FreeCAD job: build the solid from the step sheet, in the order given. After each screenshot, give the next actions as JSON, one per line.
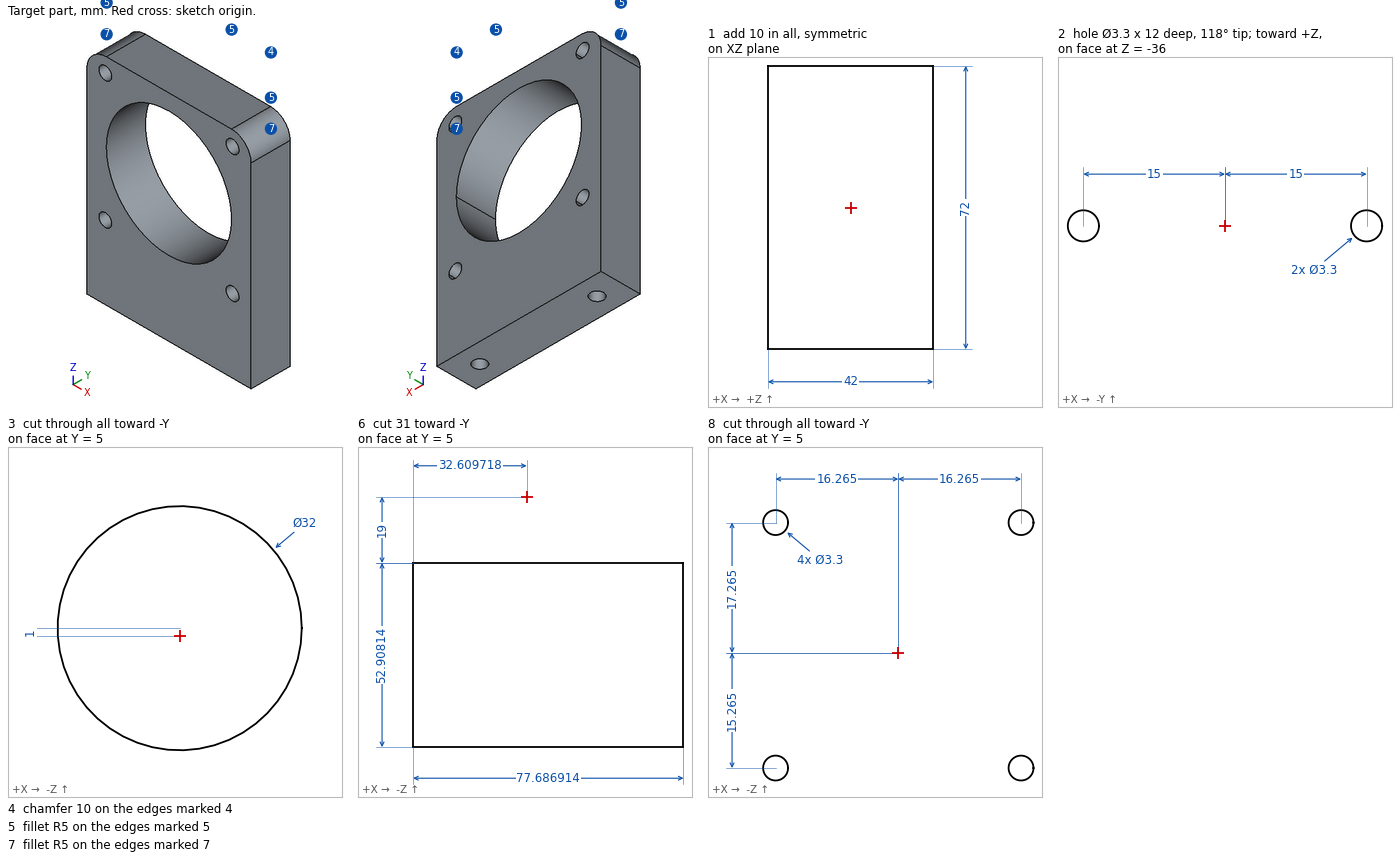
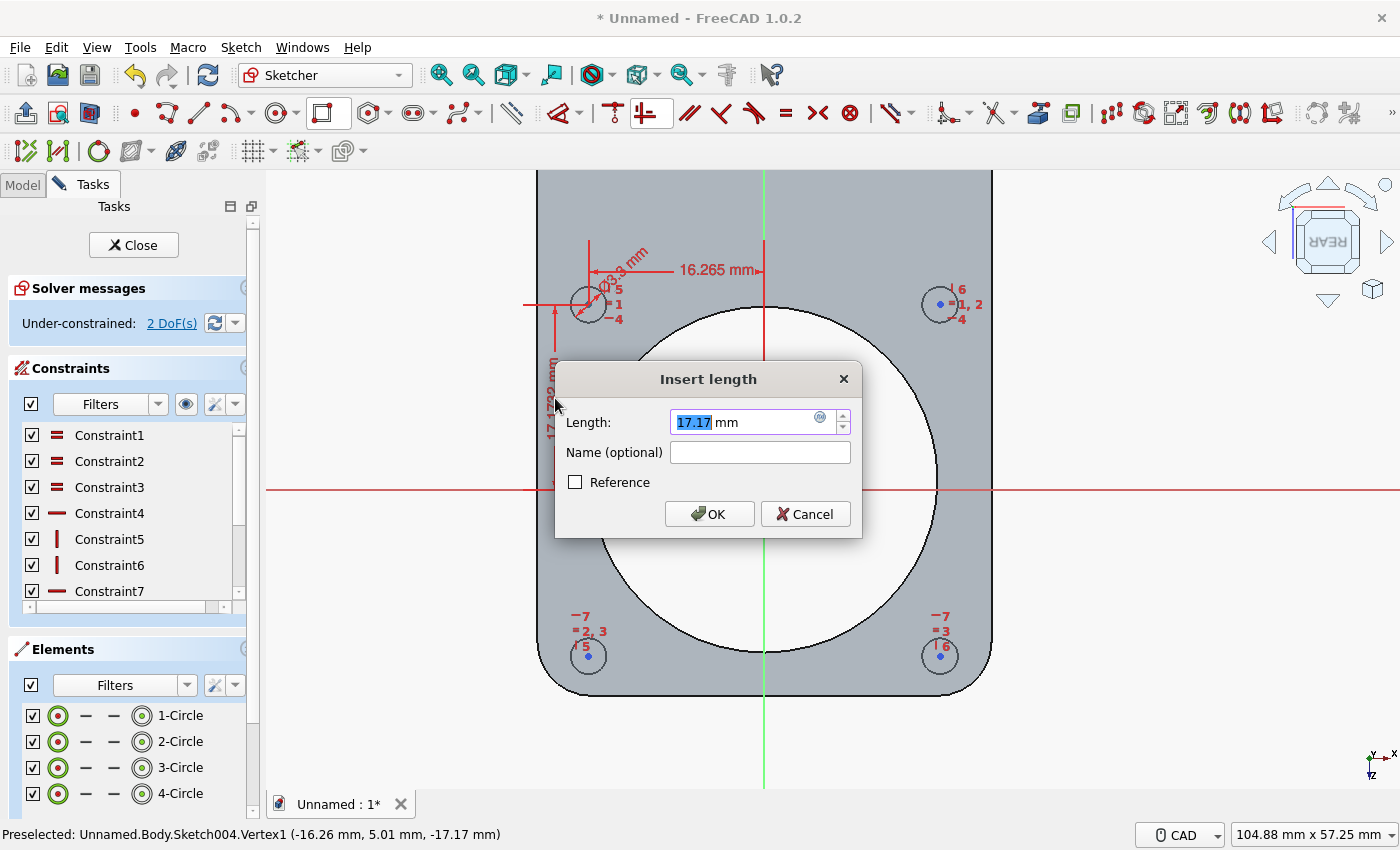
{"action": "type", "text": "17.265"}
{"action": "key", "text": "Return"}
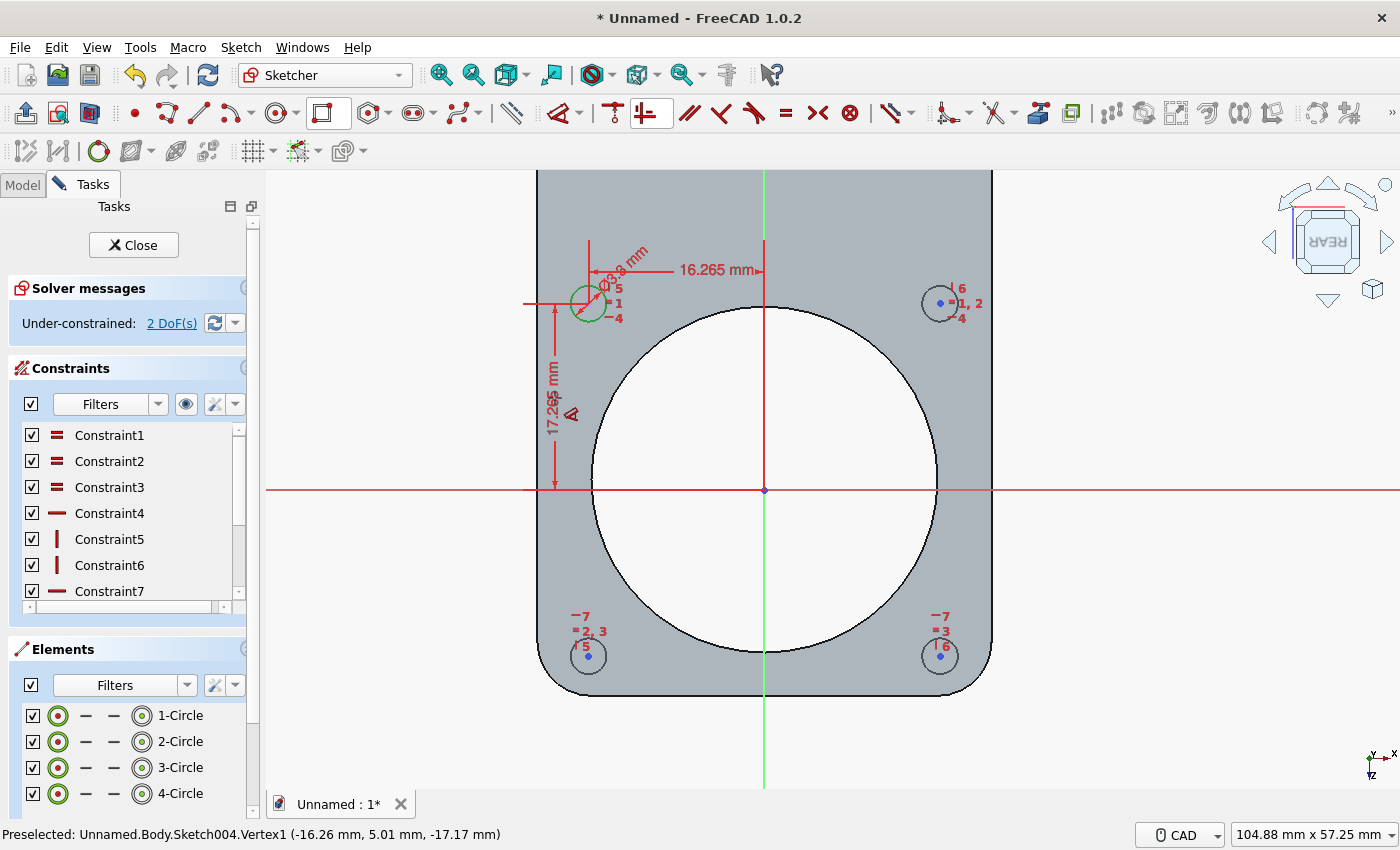
{"action": "left_click", "coordinate": [940, 304]}
{"action": "left_click", "coordinate": [852, 270]}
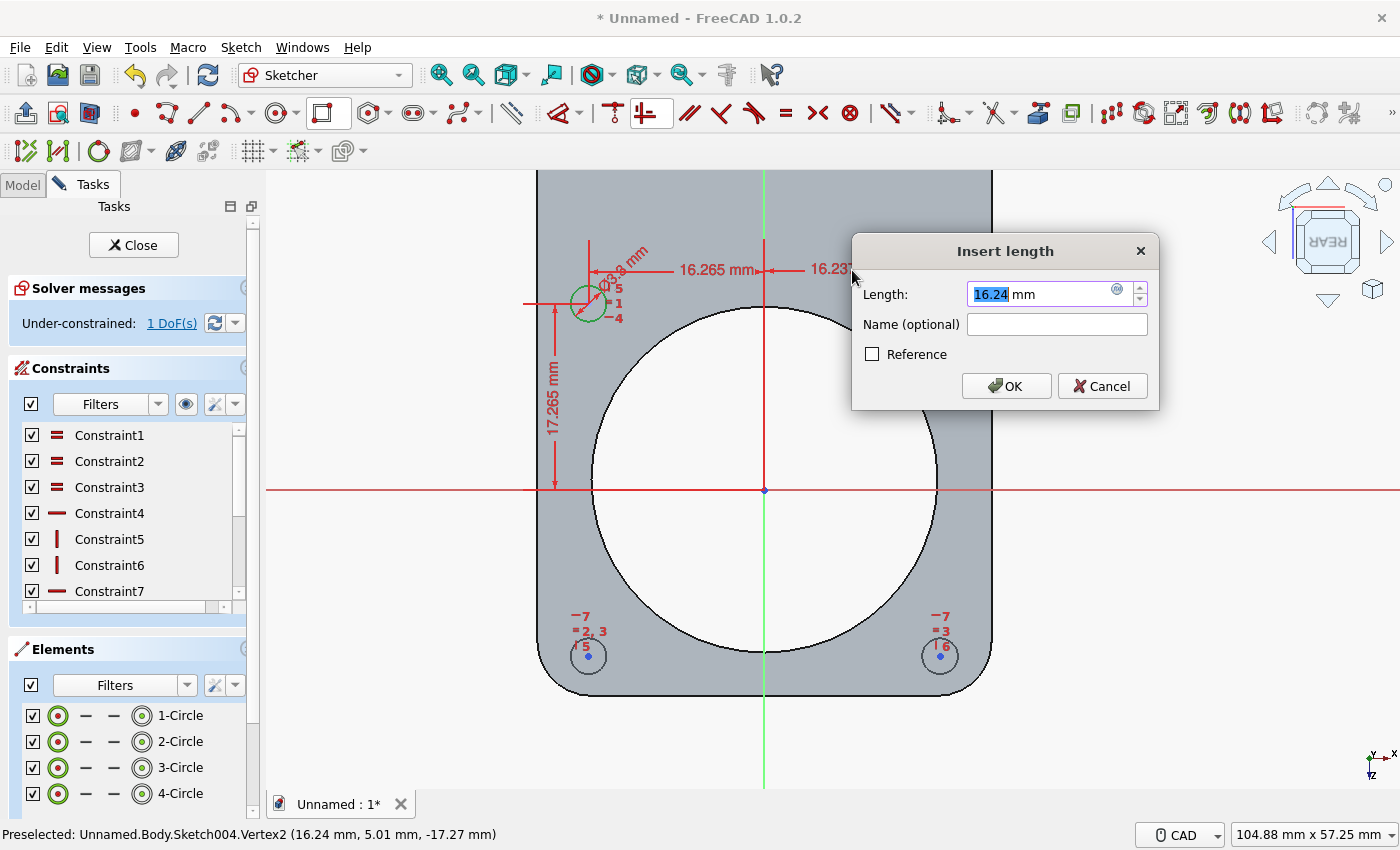
{"action": "type", "text": "16.265"}
{"action": "key", "text": "Return"}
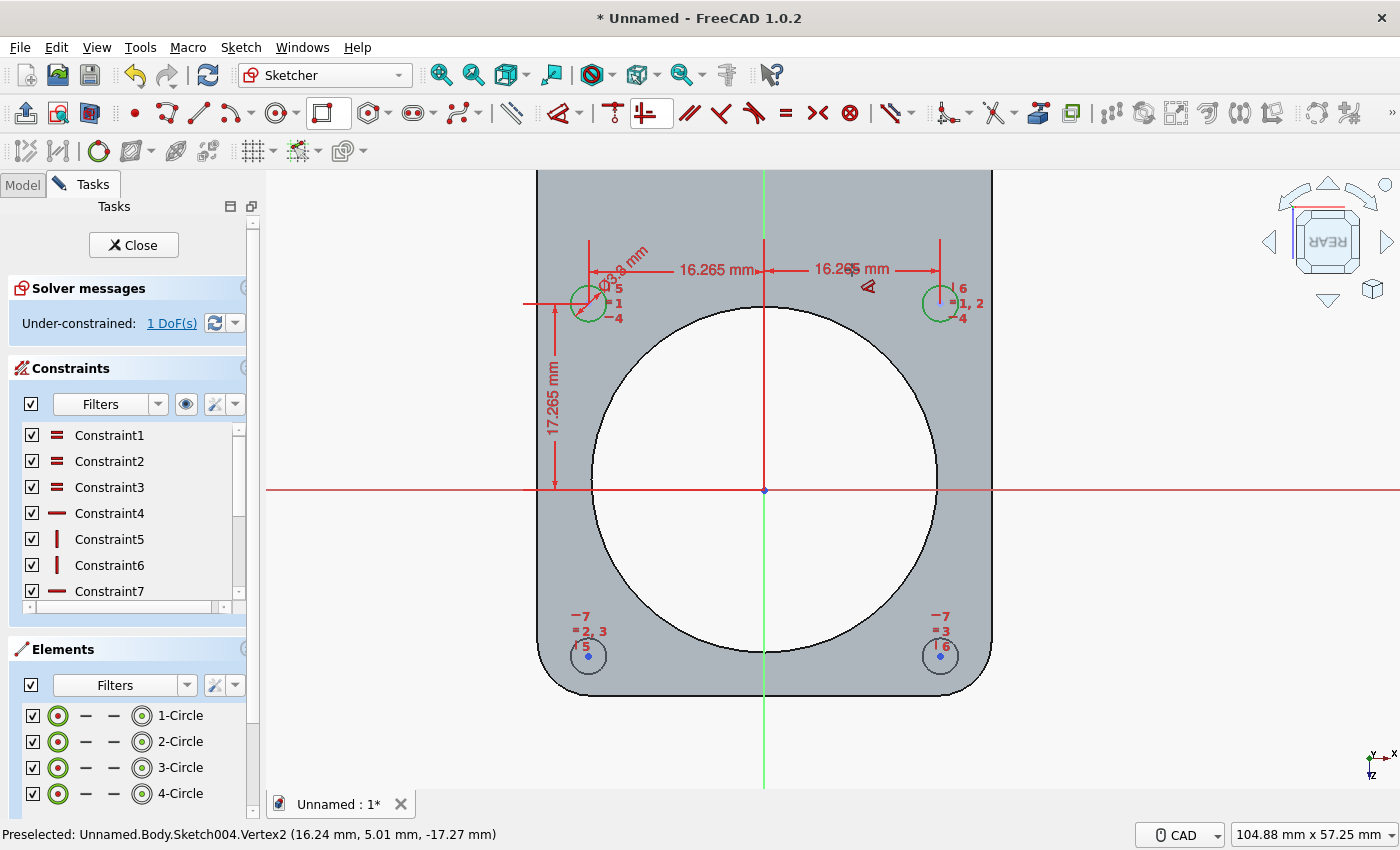
{"action": "left_click", "coordinate": [589, 656]}
{"action": "left_click", "coordinate": [555, 573]}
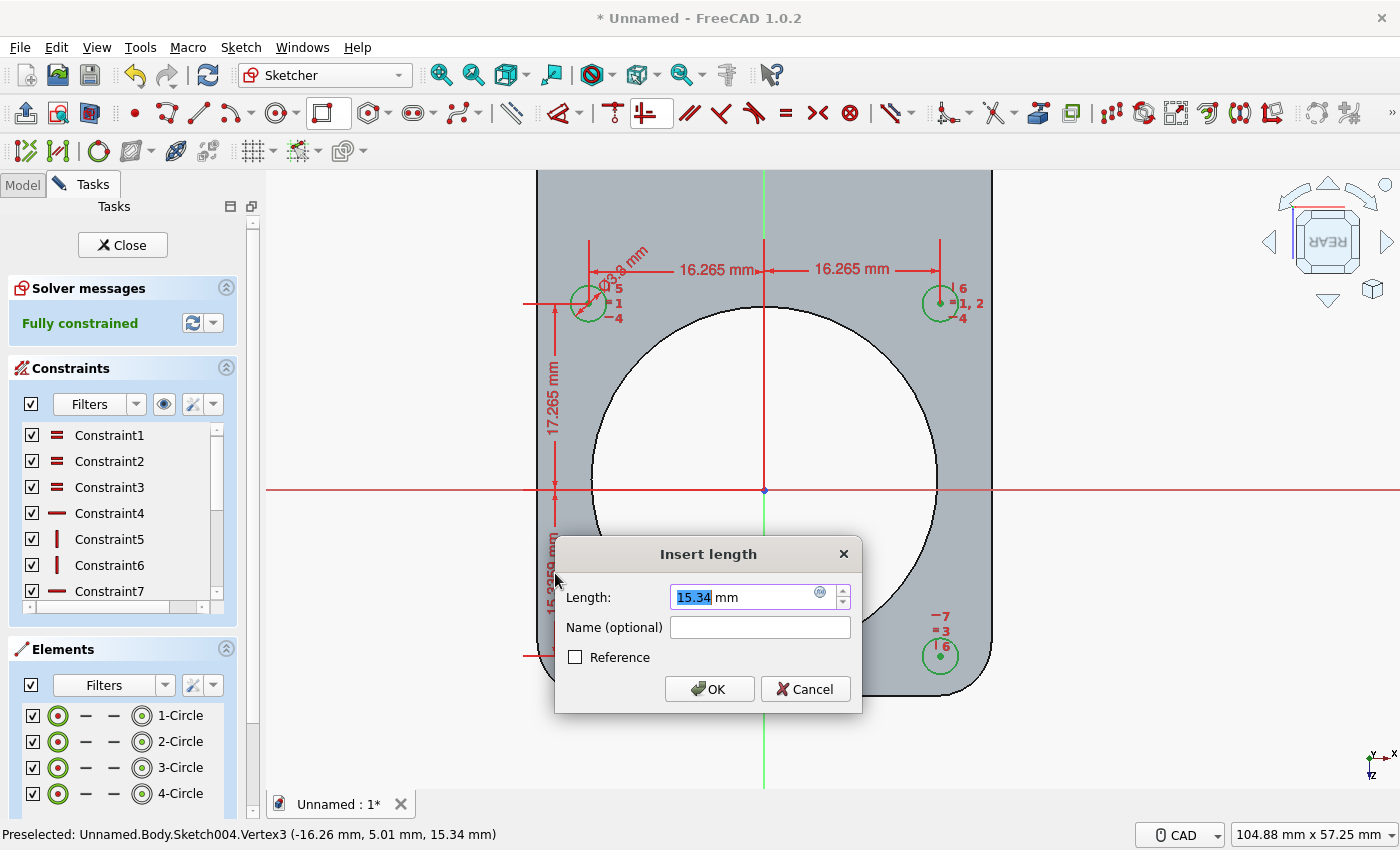
{"action": "type", "text": "15.265"}
{"action": "key", "text": "Return"}
{"action": "key", "text": "Escape"}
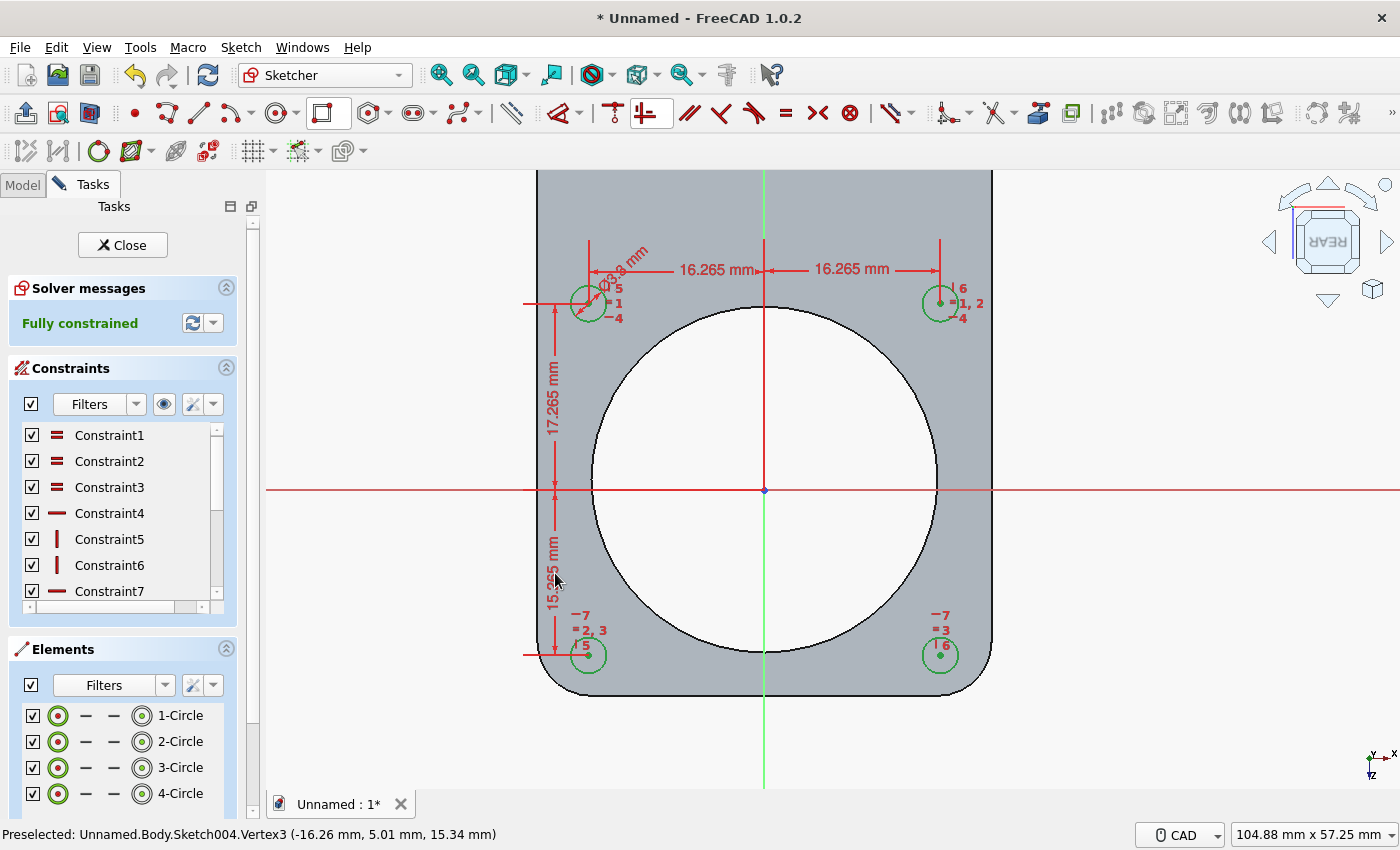
{"action": "left_click", "coordinate": [123, 245]}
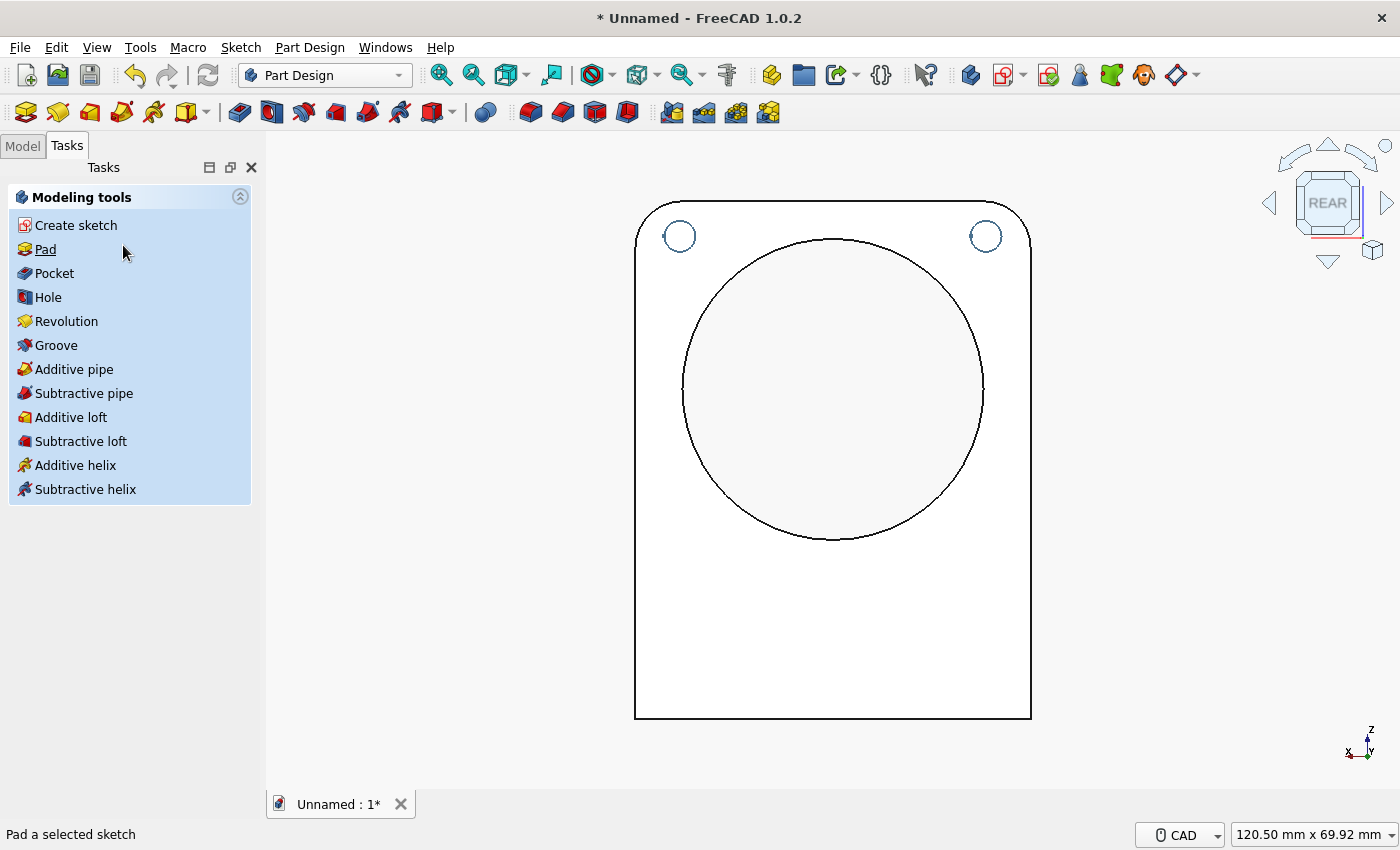
{"action": "left_click", "coordinate": [240, 112]}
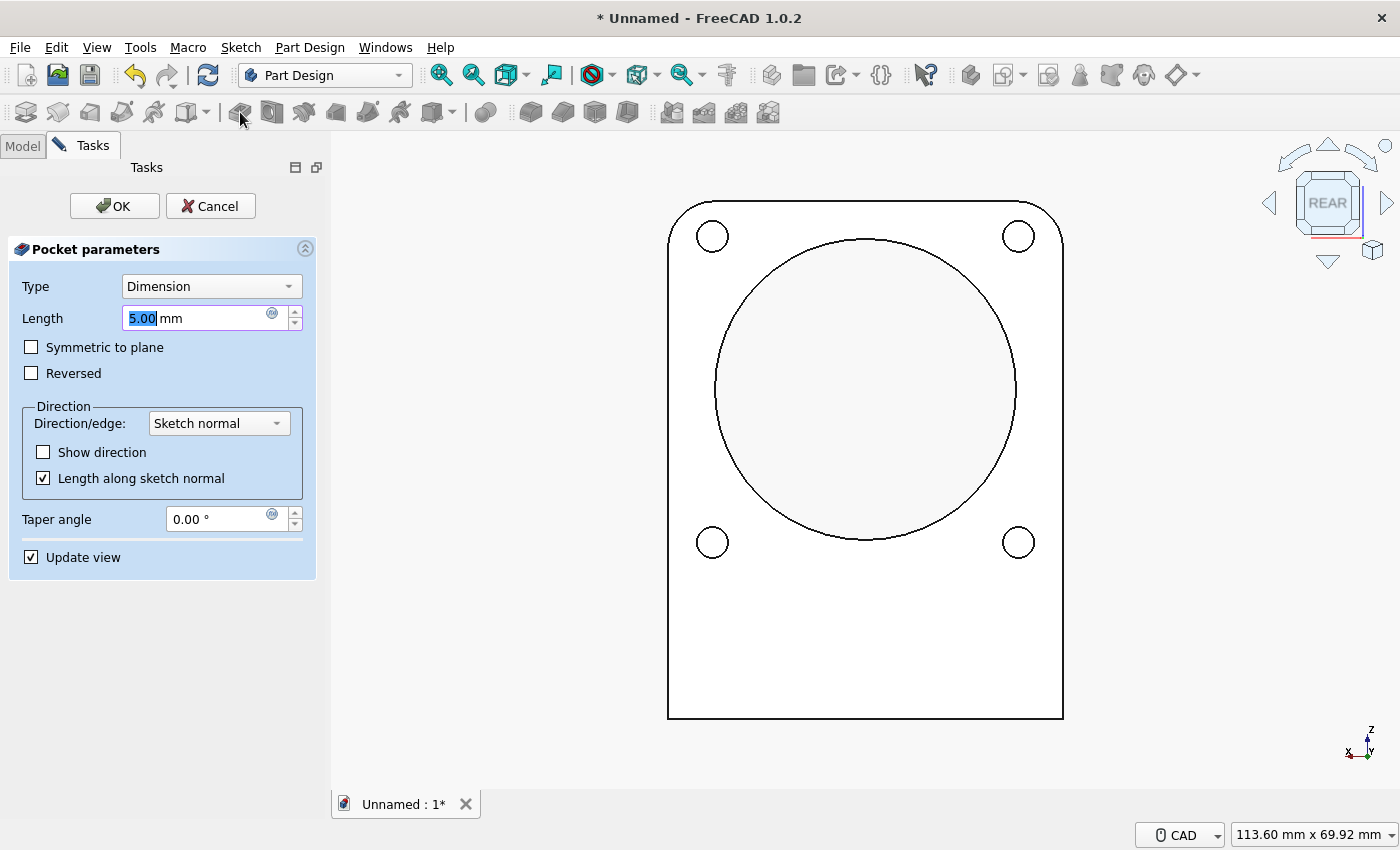
{"action": "left_click", "coordinate": [212, 286]}